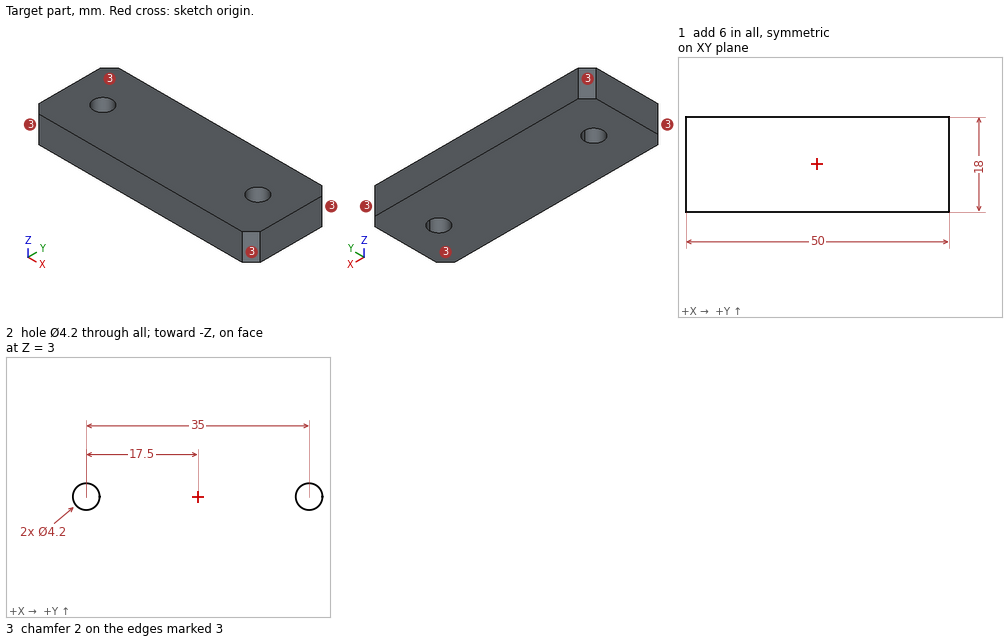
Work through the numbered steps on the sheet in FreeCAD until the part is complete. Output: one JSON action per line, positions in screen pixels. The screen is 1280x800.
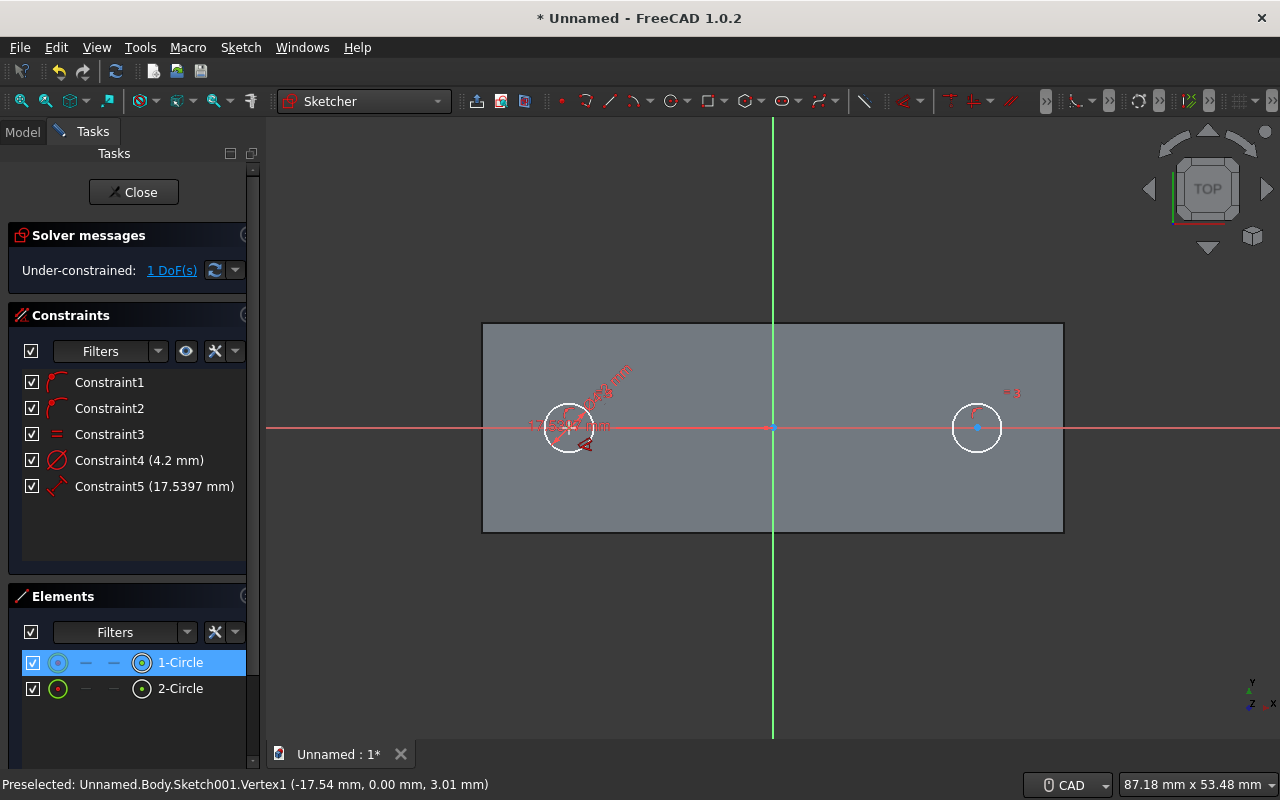
{"action": "left_click", "coordinate": [977, 428]}
{"action": "left_click", "coordinate": [679, 462]}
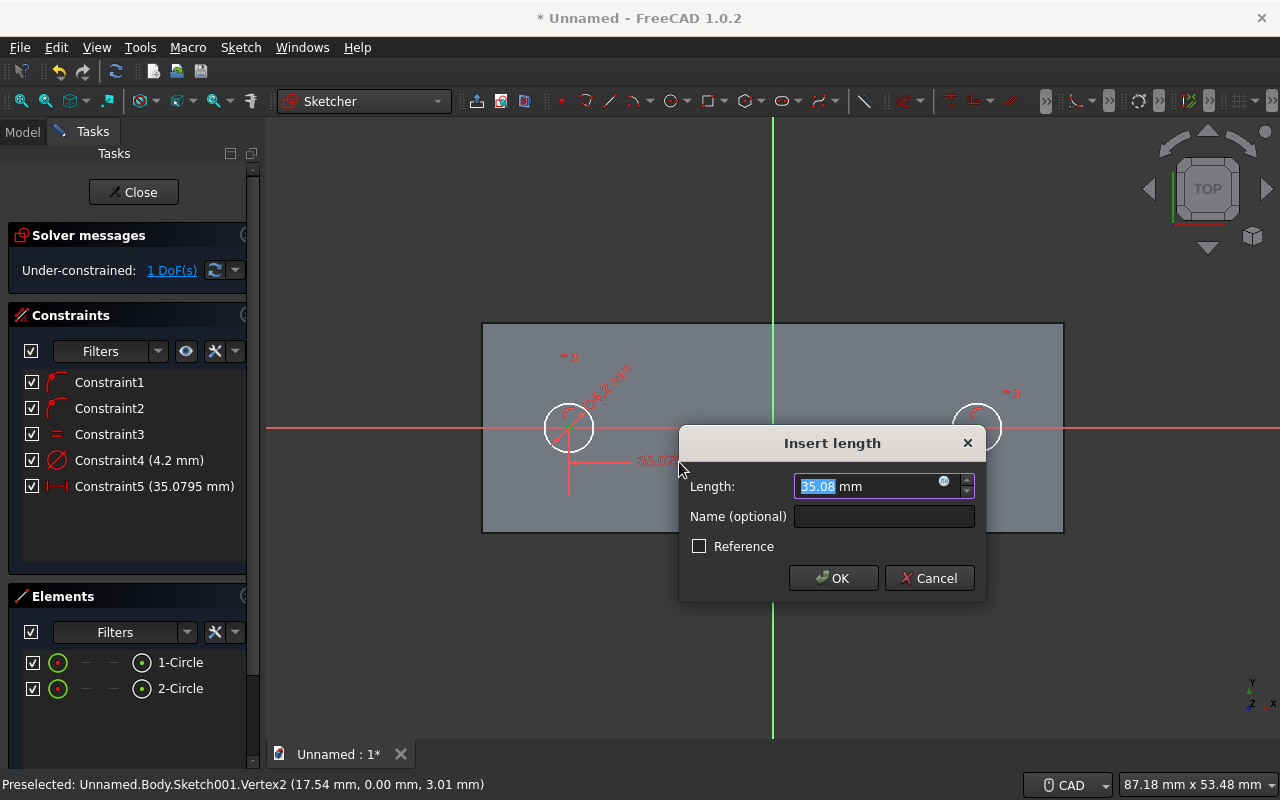
{"action": "type", "text": "35"}
{"action": "key", "text": "Return"}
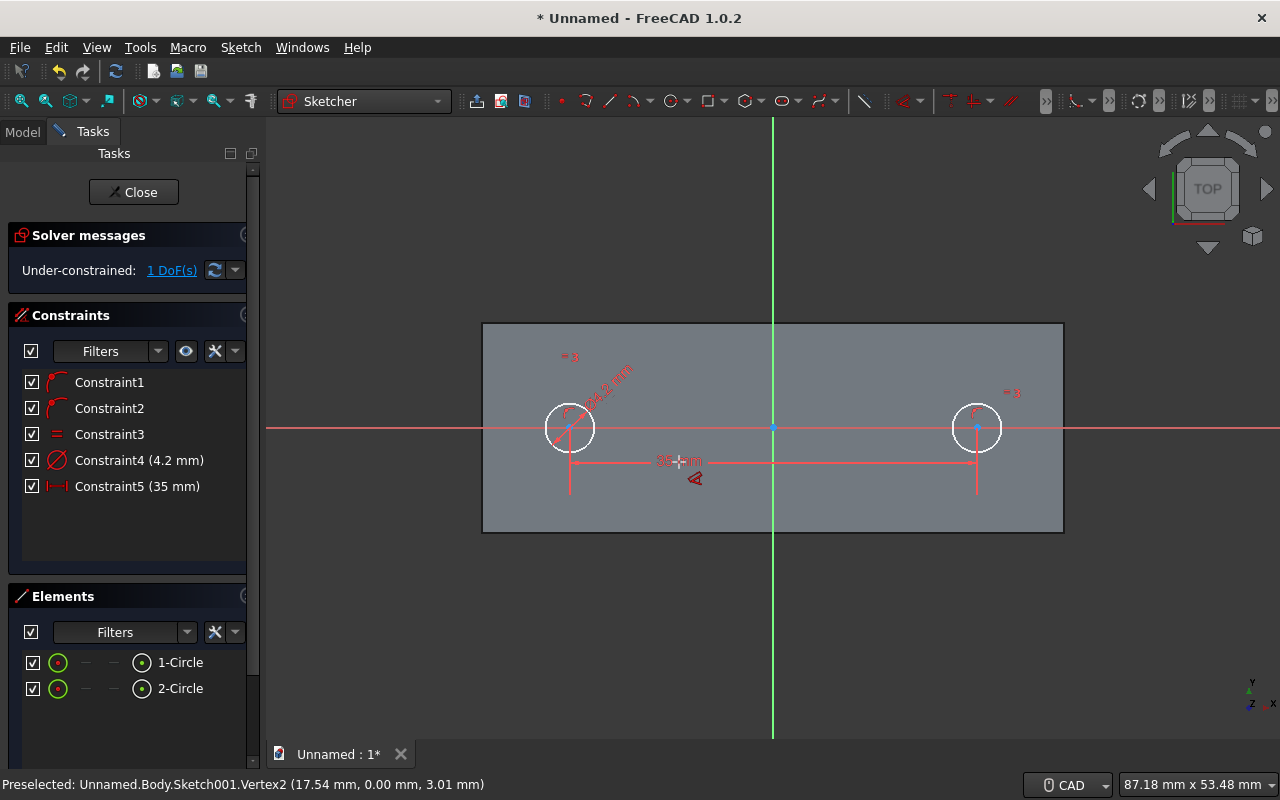
{"action": "left_click", "coordinate": [570, 428]}
{"action": "left_click", "coordinate": [600, 462]}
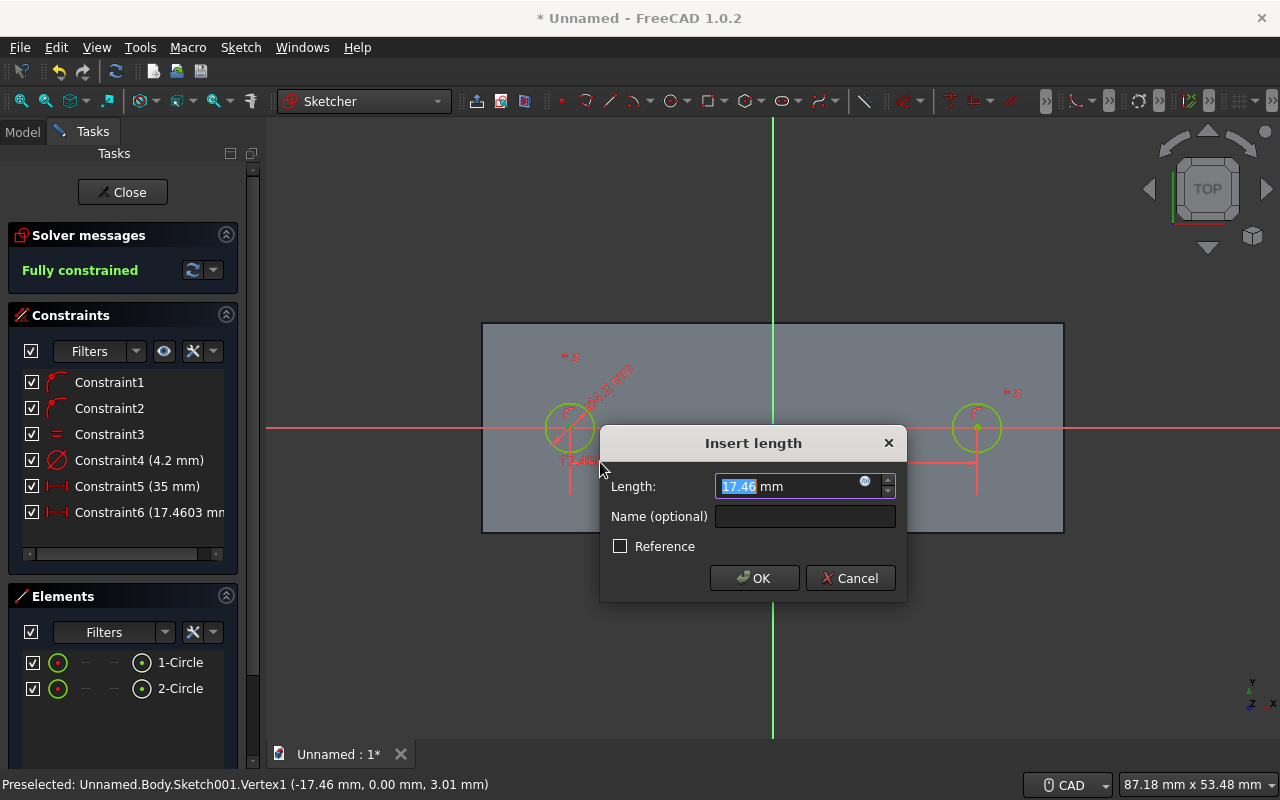
{"action": "type", "text": "17.5"}
{"action": "key", "text": "Return"}
{"action": "key", "text": "Escape"}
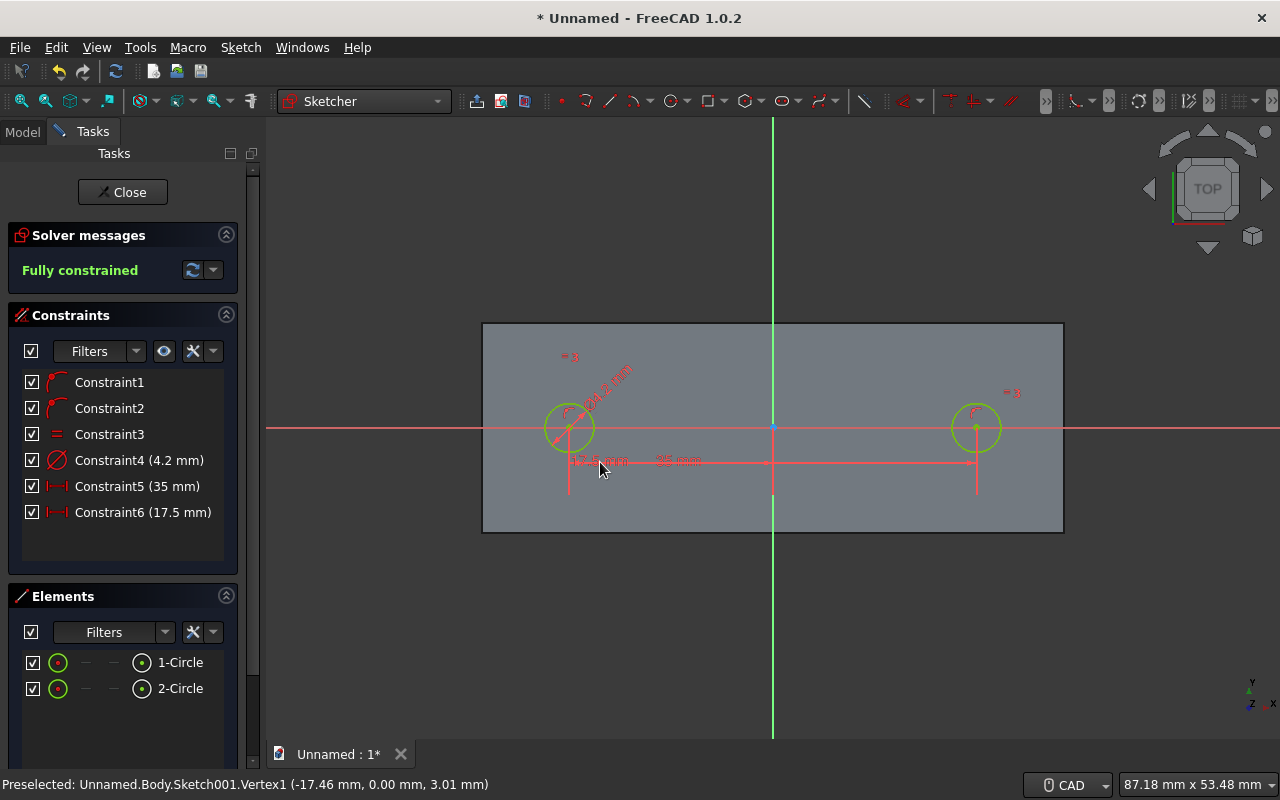
{"action": "left_click", "coordinate": [123, 192]}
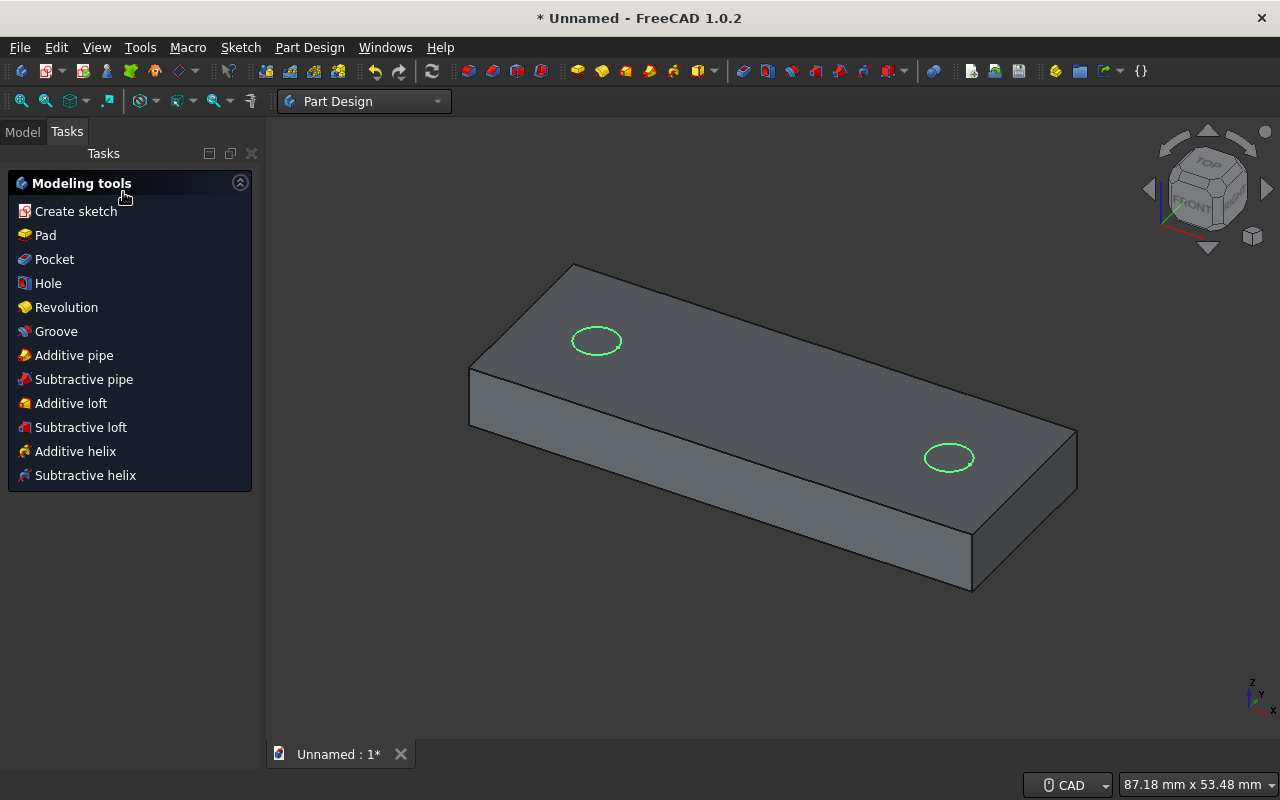
{"action": "left_click", "coordinate": [768, 72]}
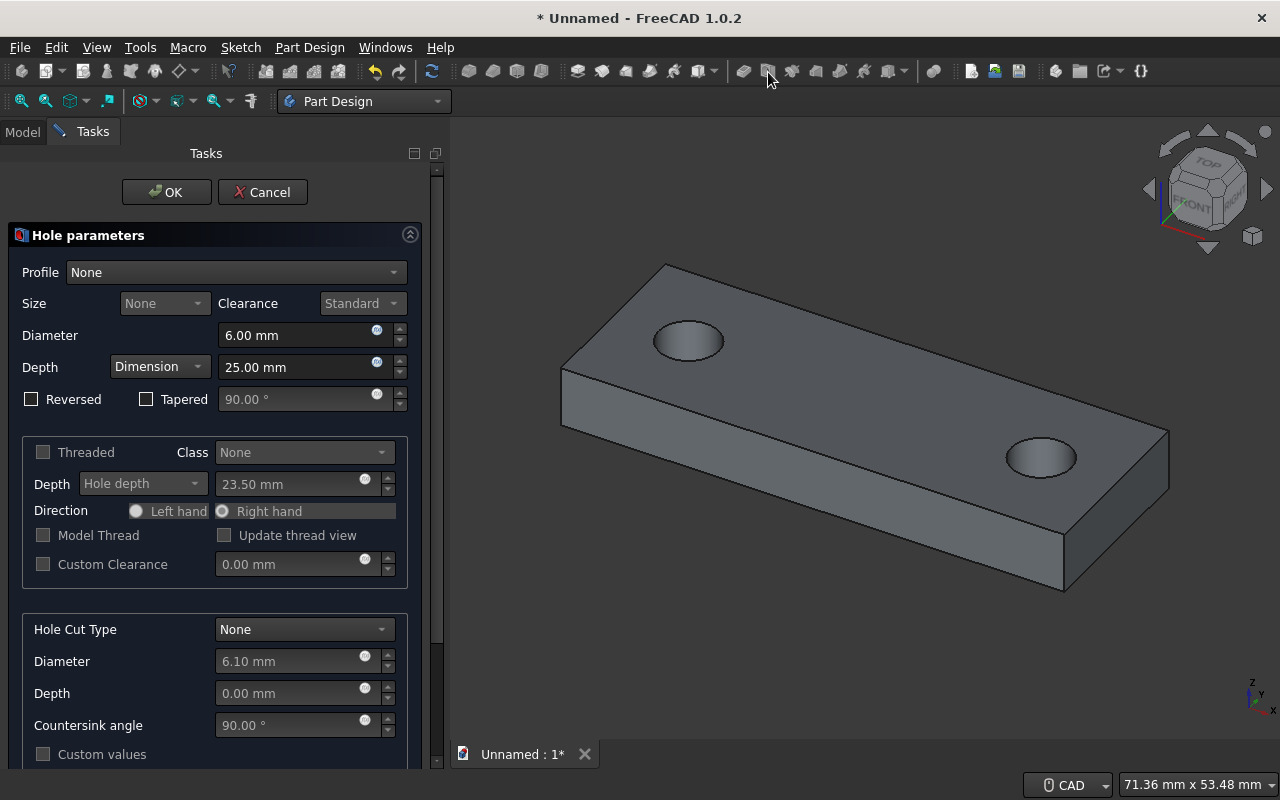
{"action": "triple_click", "coordinate": [305, 335]}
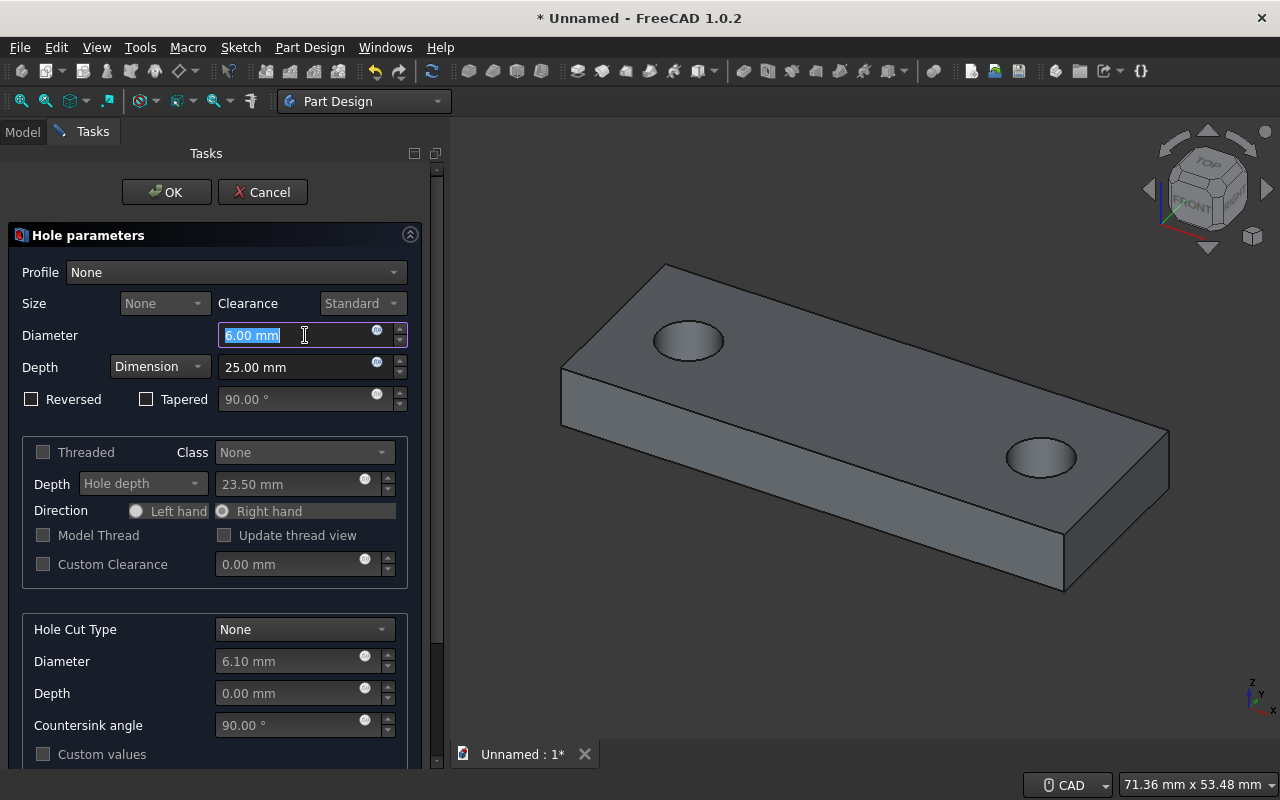
{"action": "type", "text": "4.2"}
{"action": "key", "text": "Tab"}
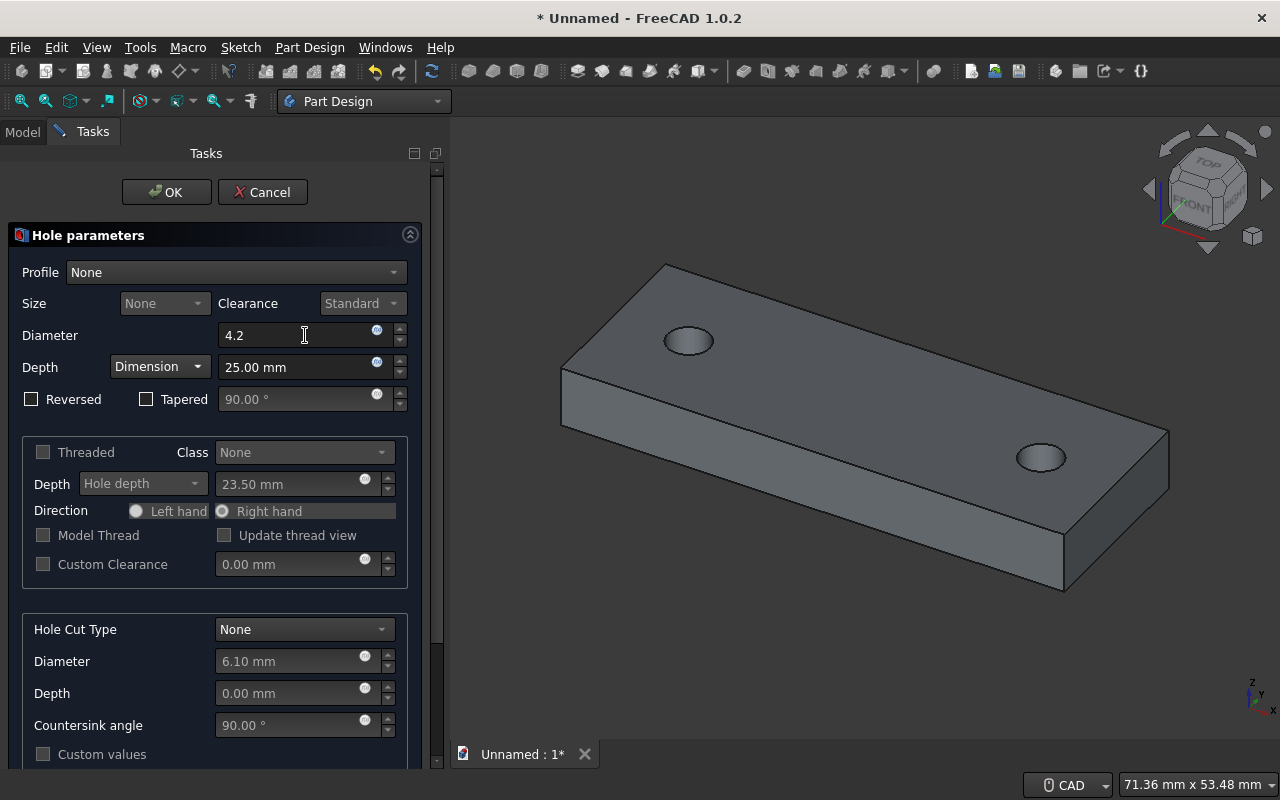
{"action": "left_click", "coordinate": [161, 366]}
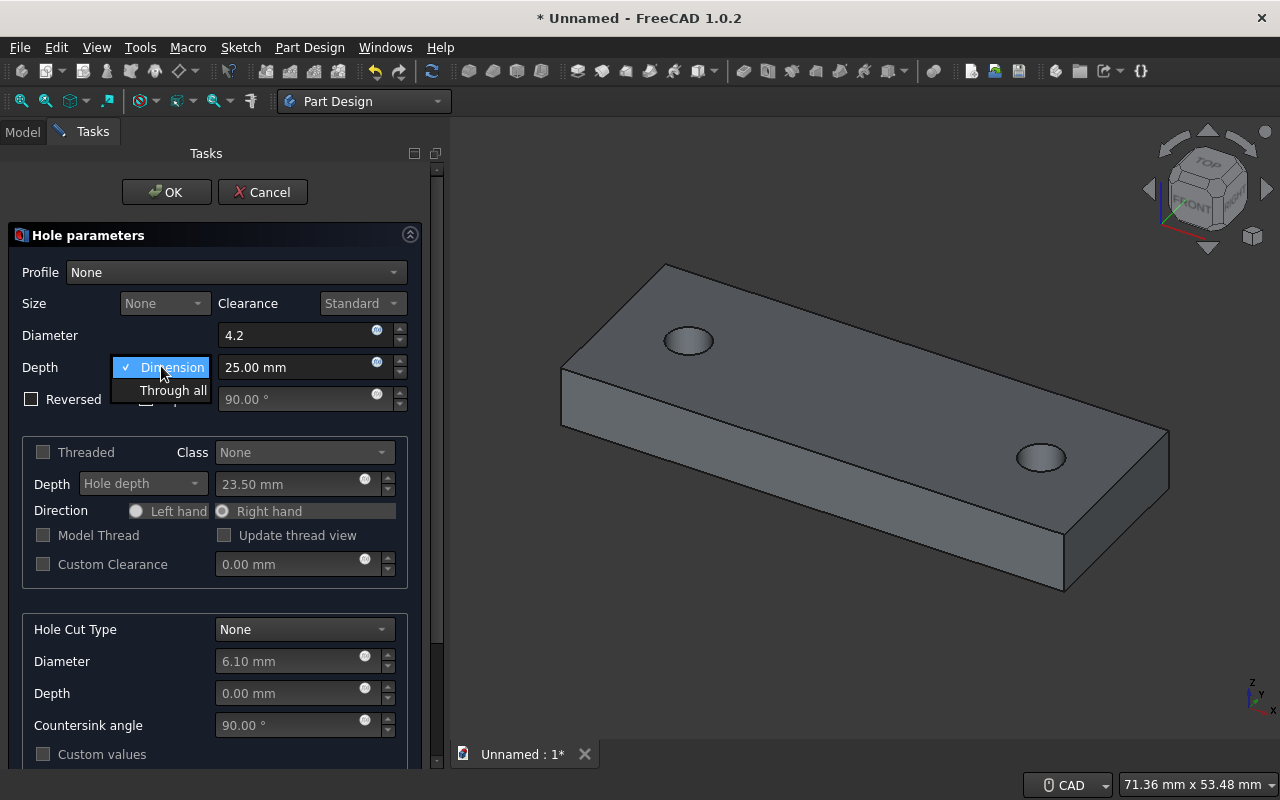
{"action": "left_click", "coordinate": [160, 390]}